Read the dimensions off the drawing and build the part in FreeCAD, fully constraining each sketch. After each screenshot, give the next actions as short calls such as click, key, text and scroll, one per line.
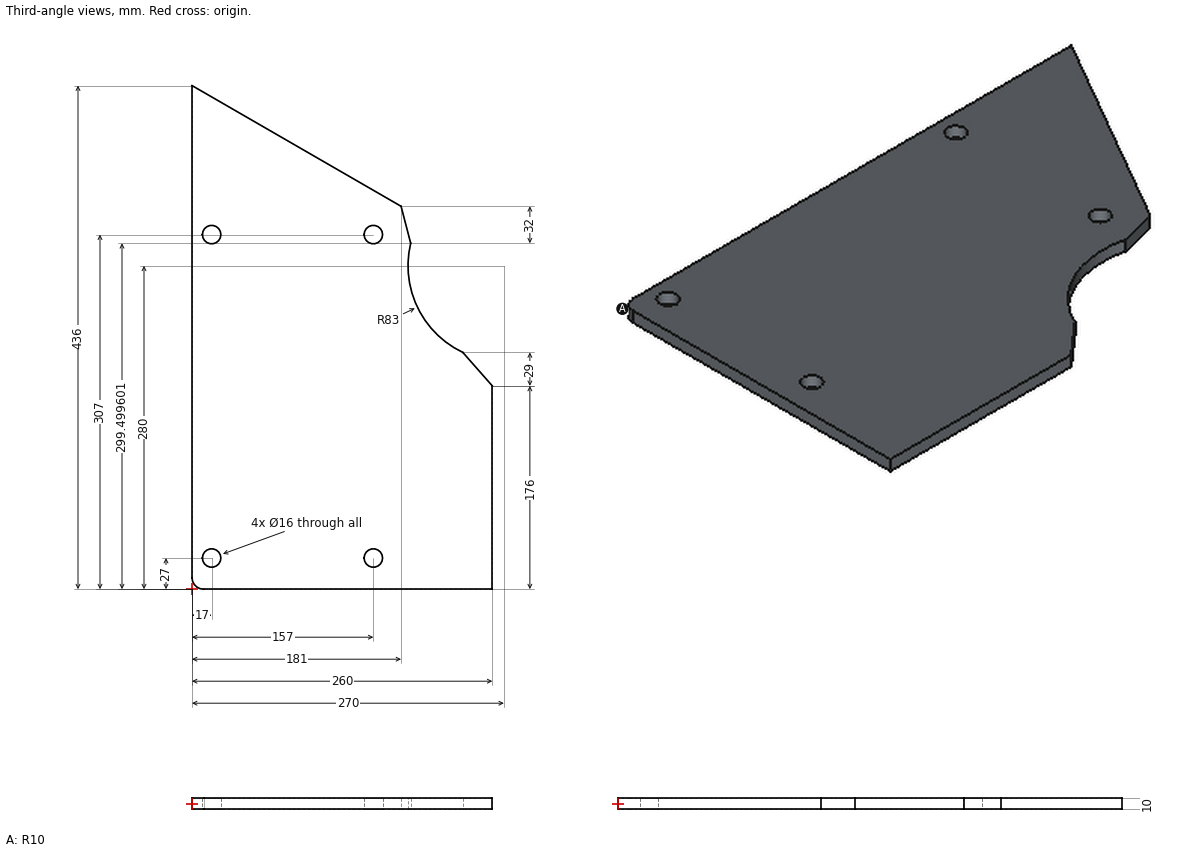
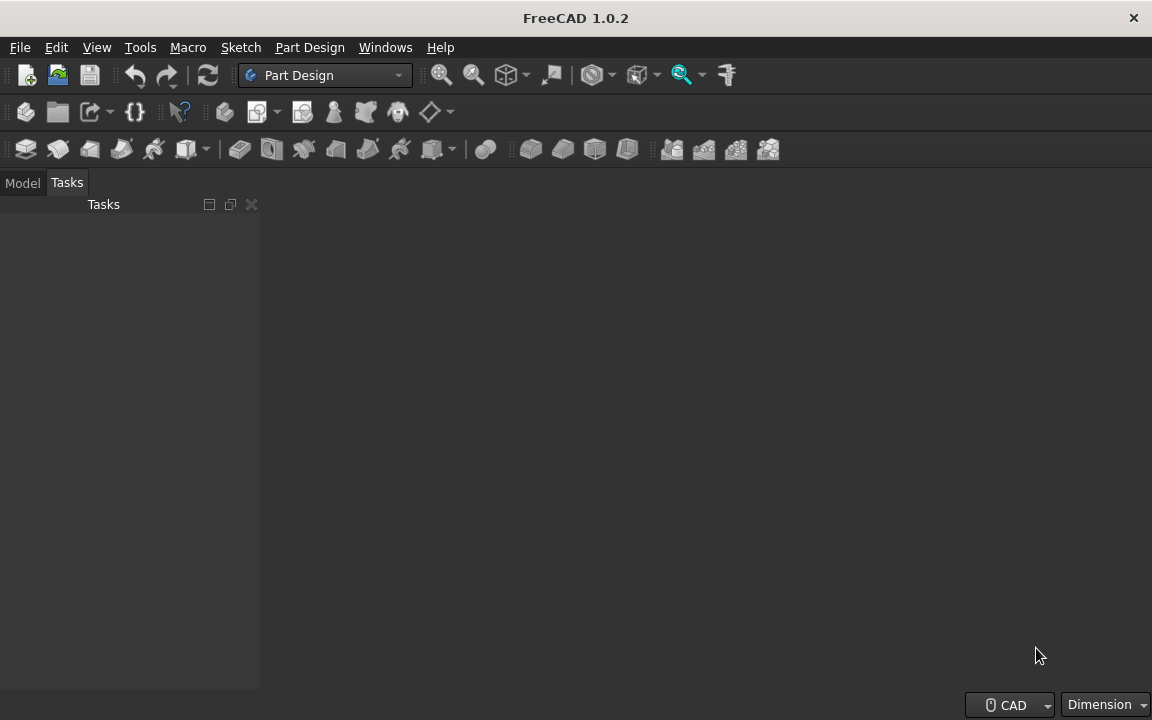
key(ctrl+n)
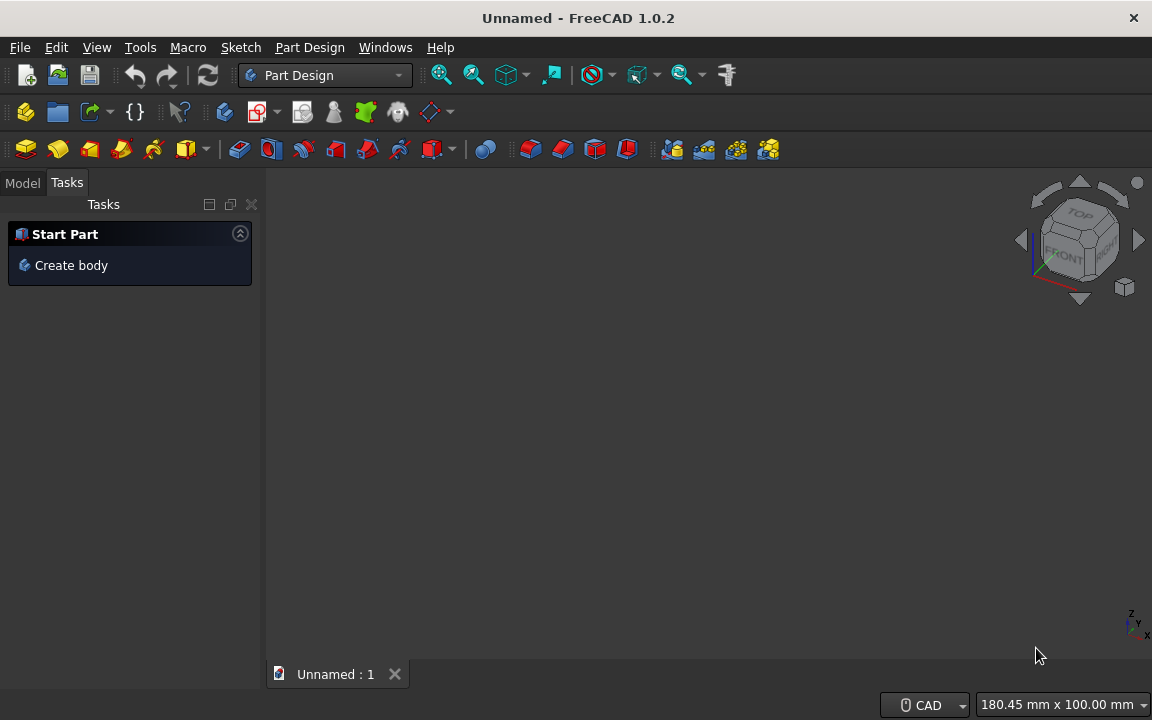
click(258, 112)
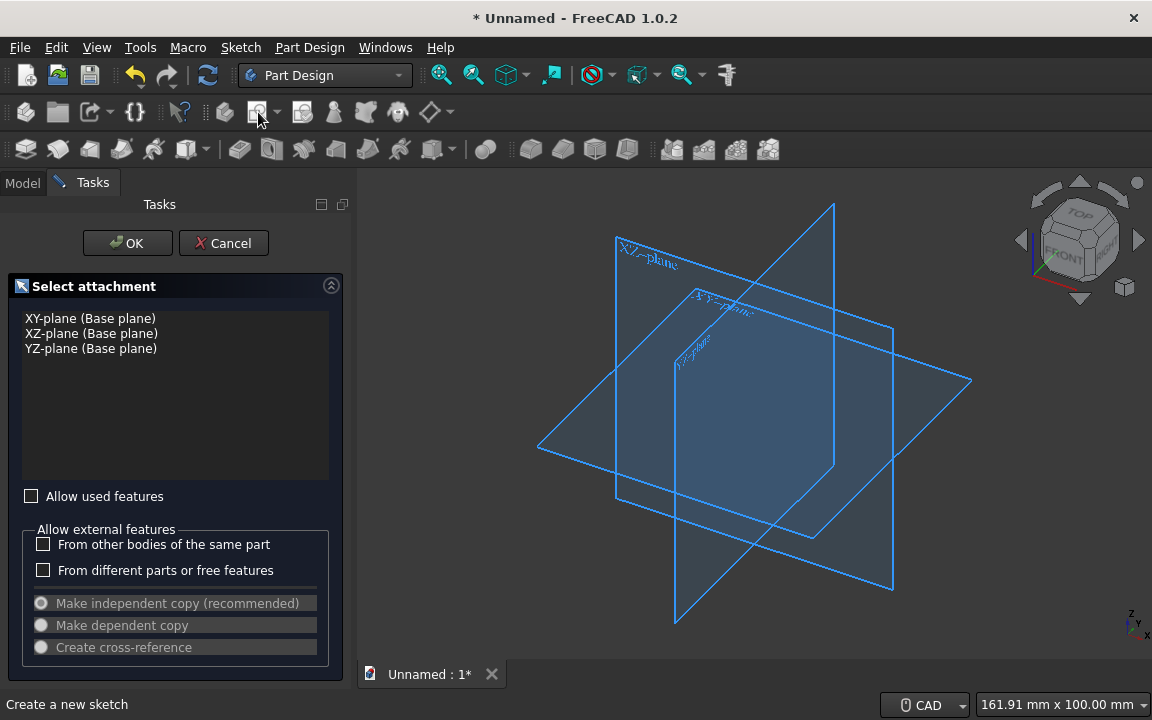
click(82, 318)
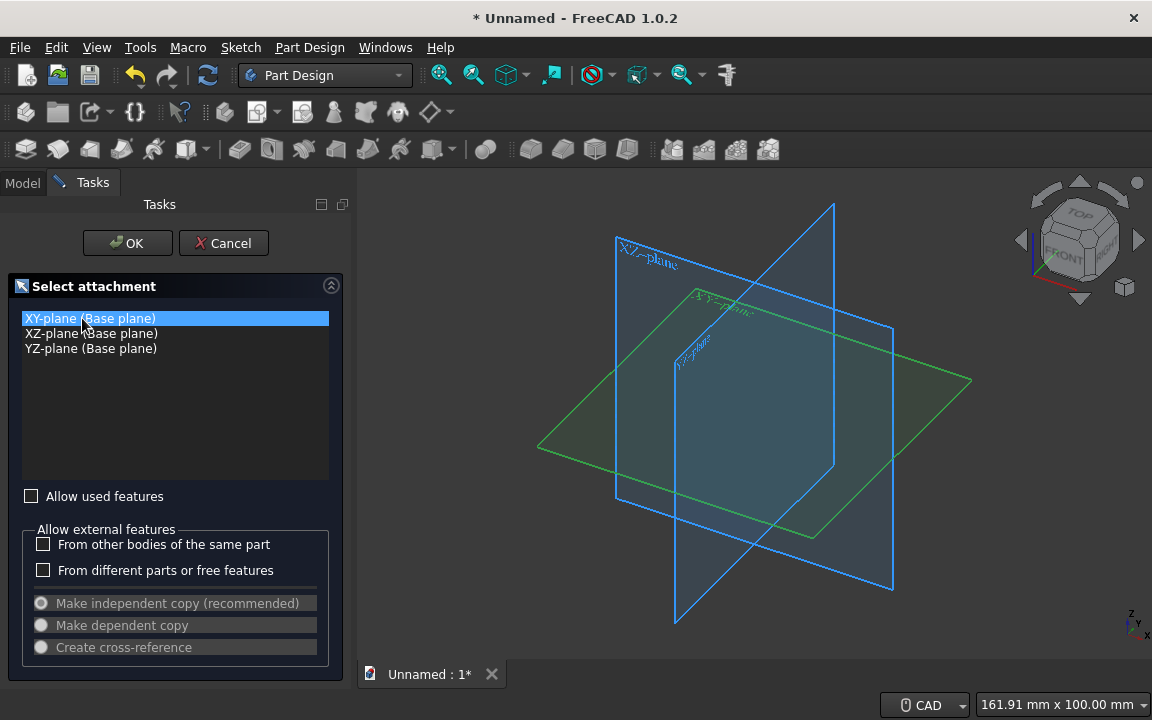
click(128, 243)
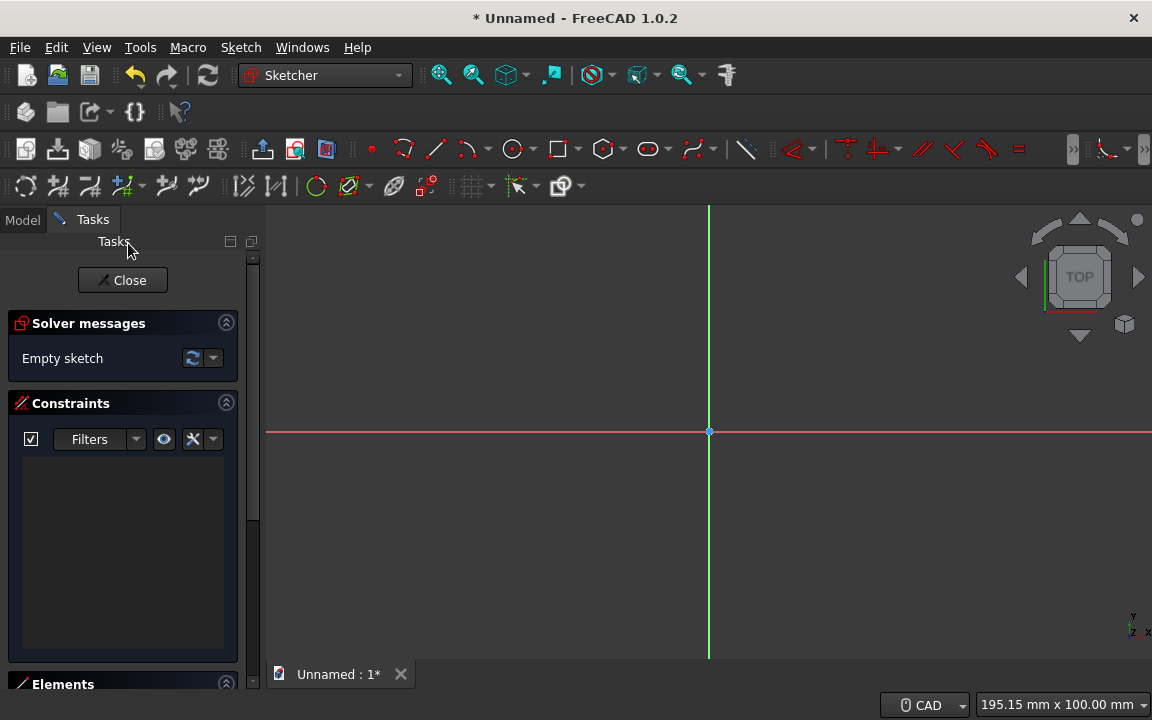
scroll(537, 587, down, 10)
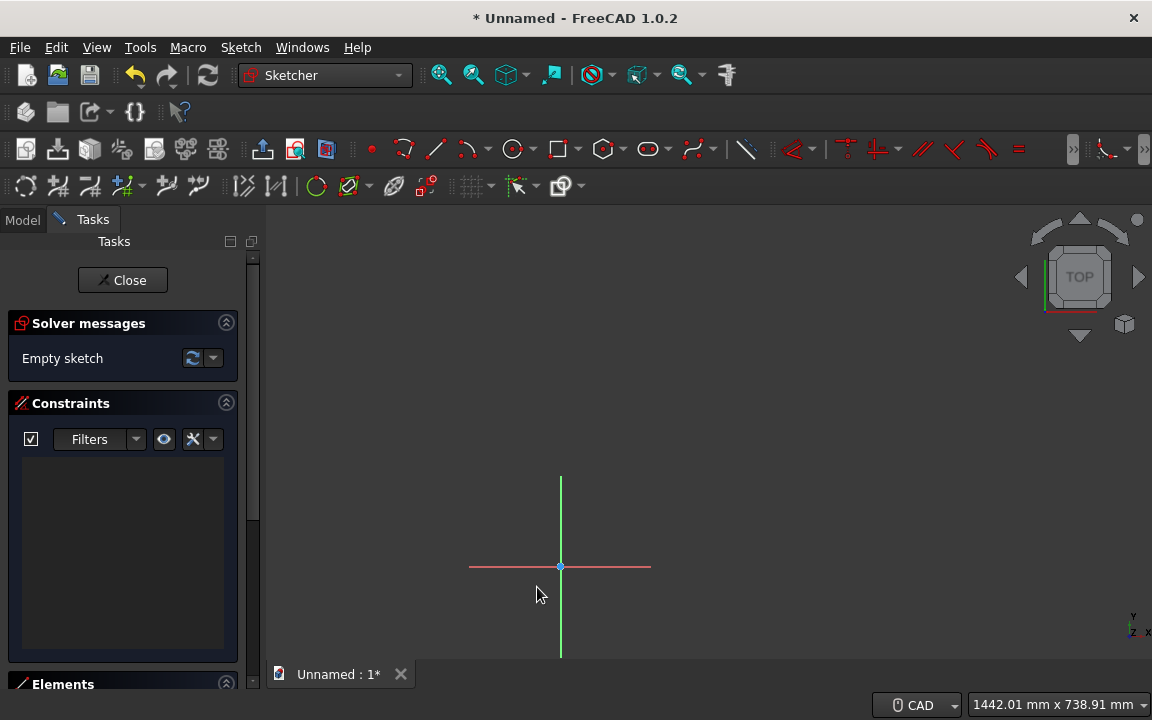
click(404, 150)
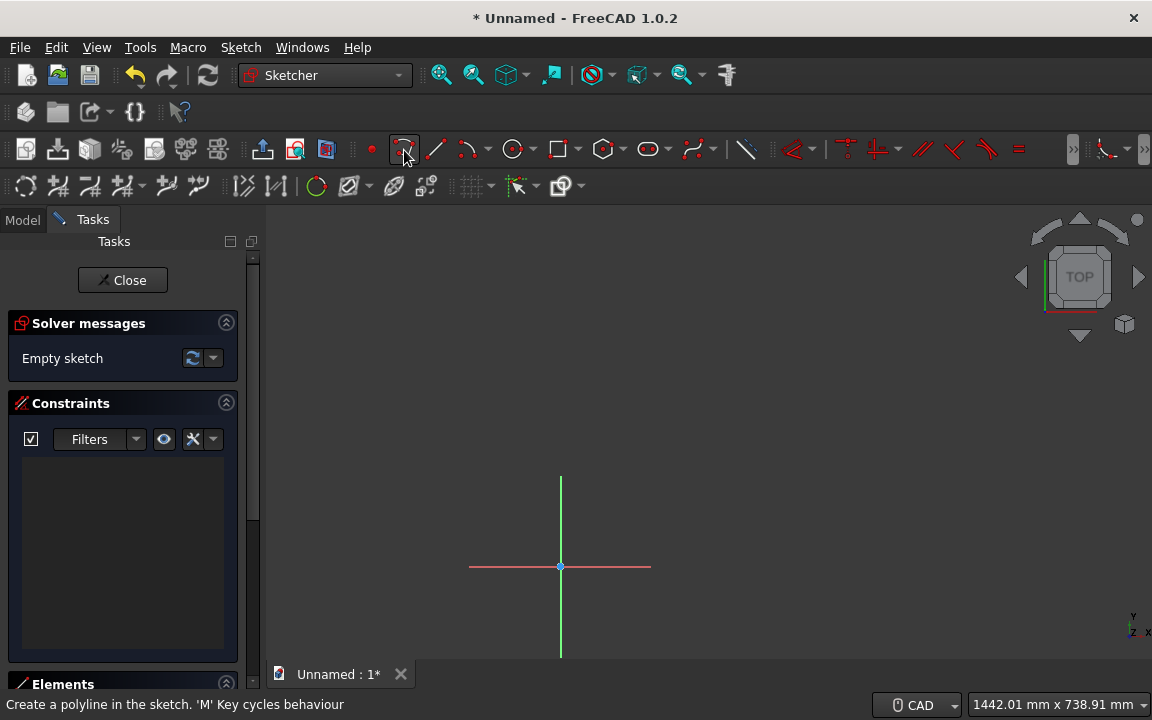
click(677, 383)
click(672, 363)
click(561, 299)
click(561, 567)
click(720, 558)
click(720, 459)
click(705, 441)
right_click(705, 441)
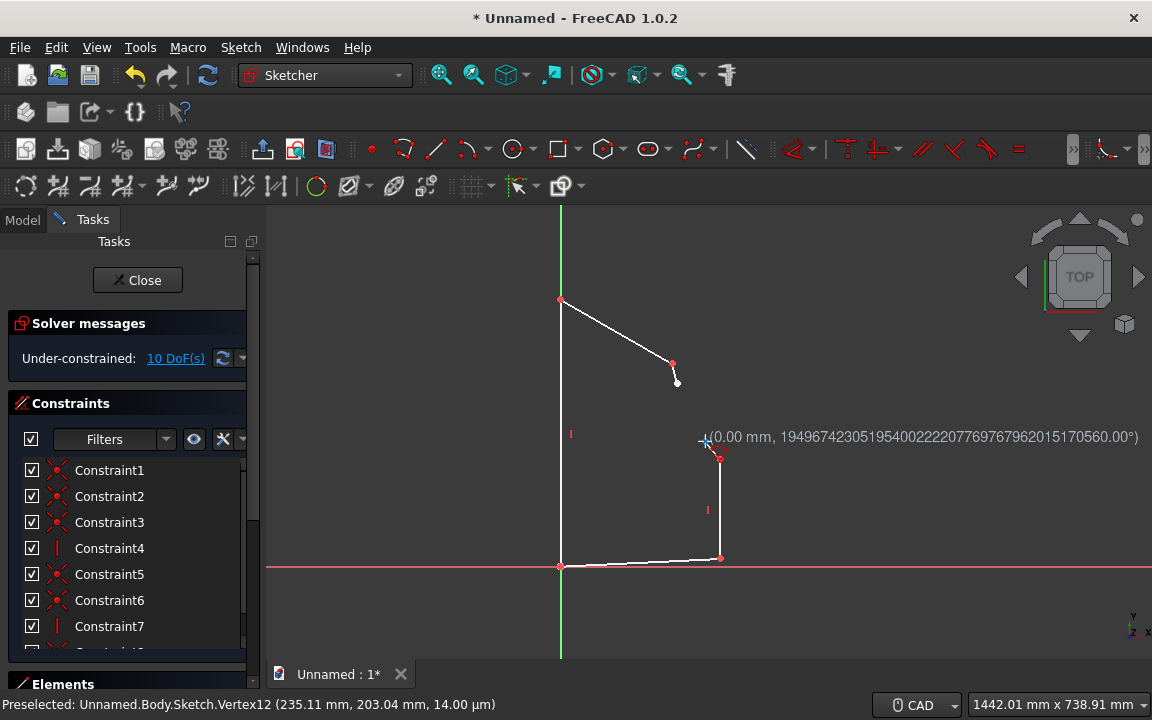
key(g)
key(3)
key(a)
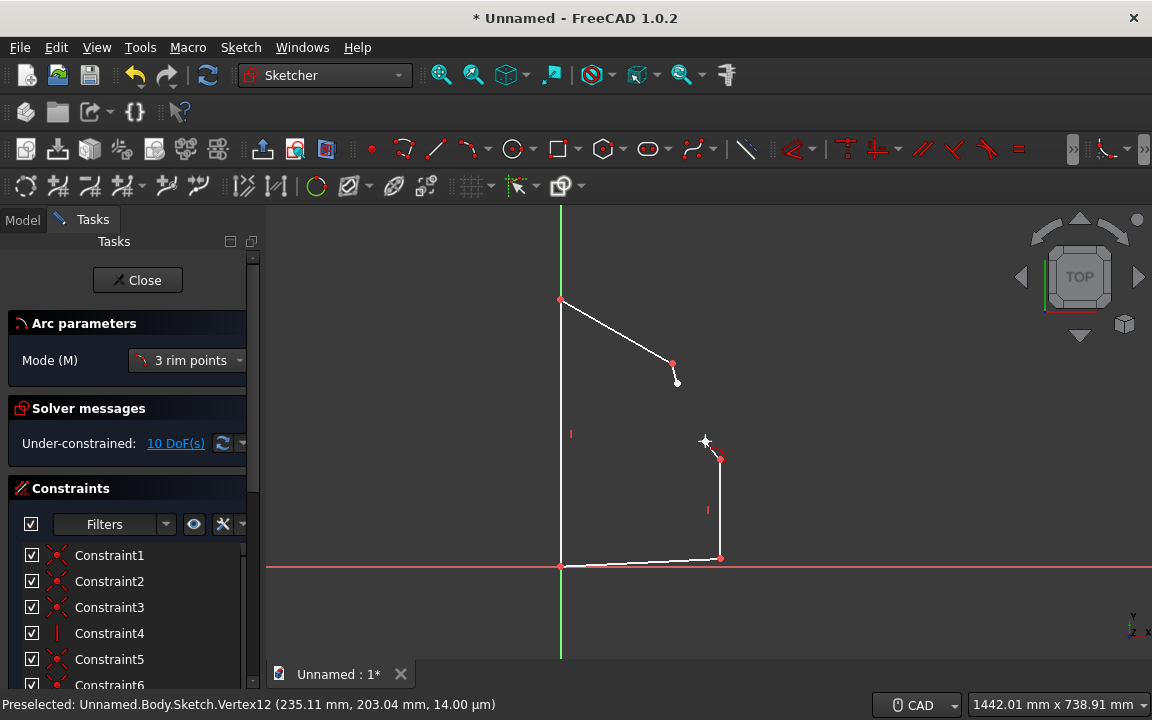
scroll(705, 441, up, 2)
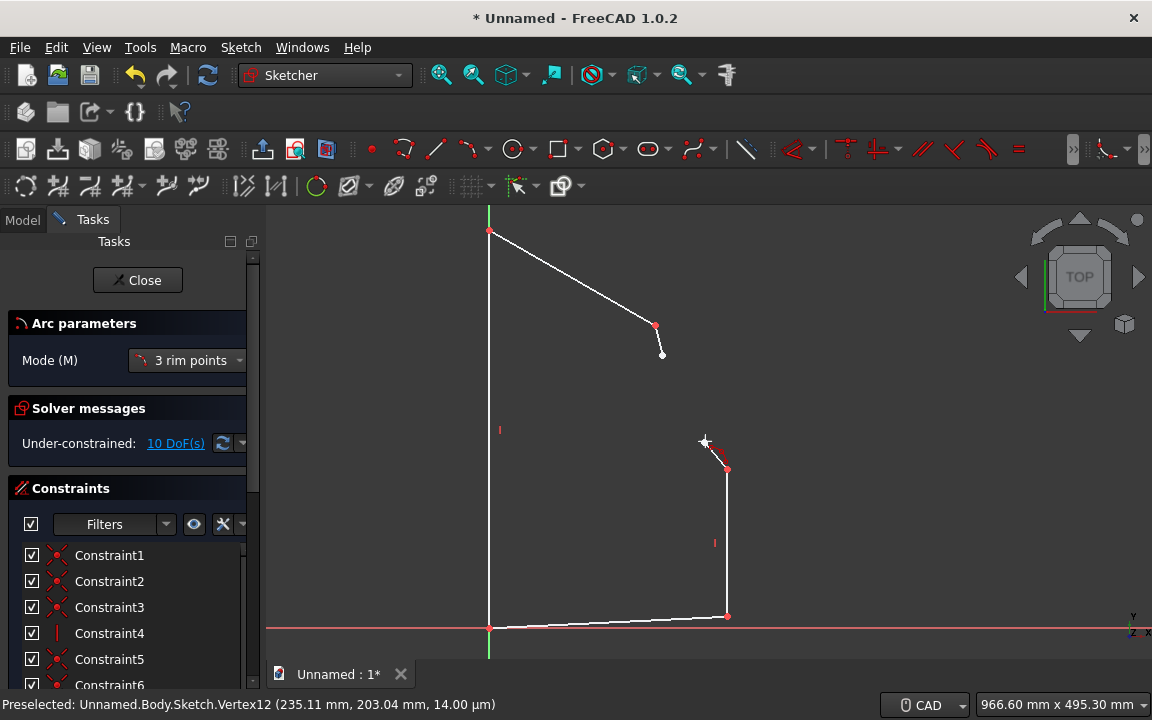
click(705, 442)
click(663, 356)
click(668, 404)
key(Escape)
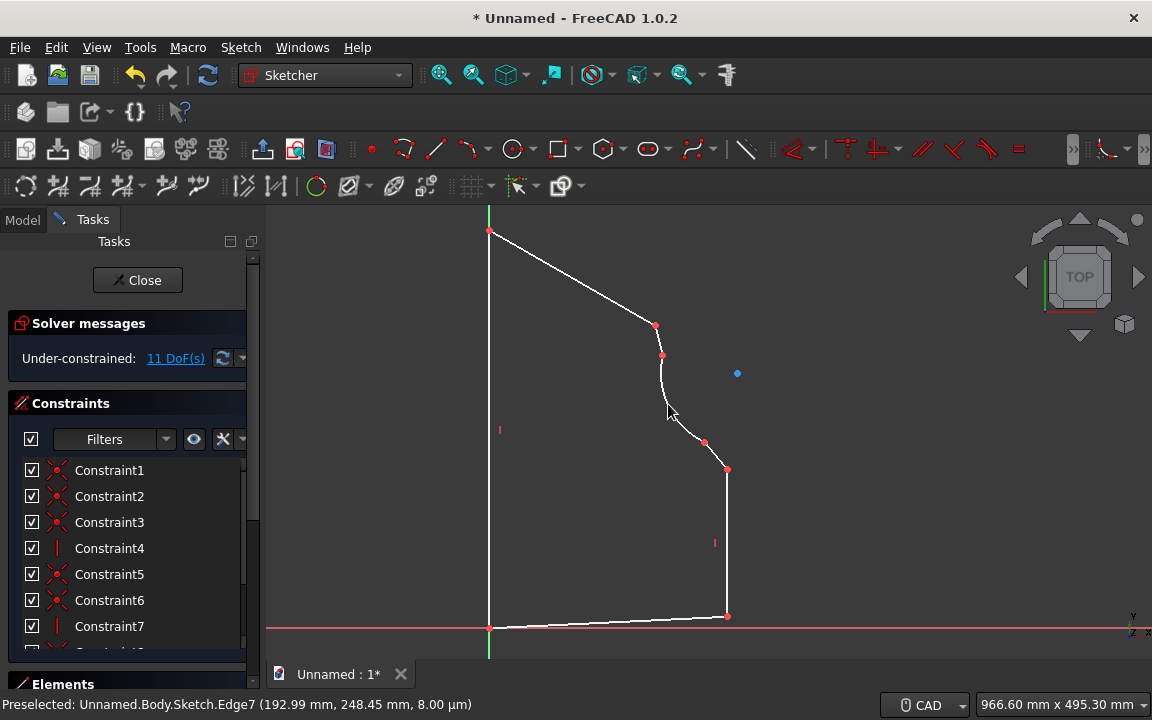
click(561, 625)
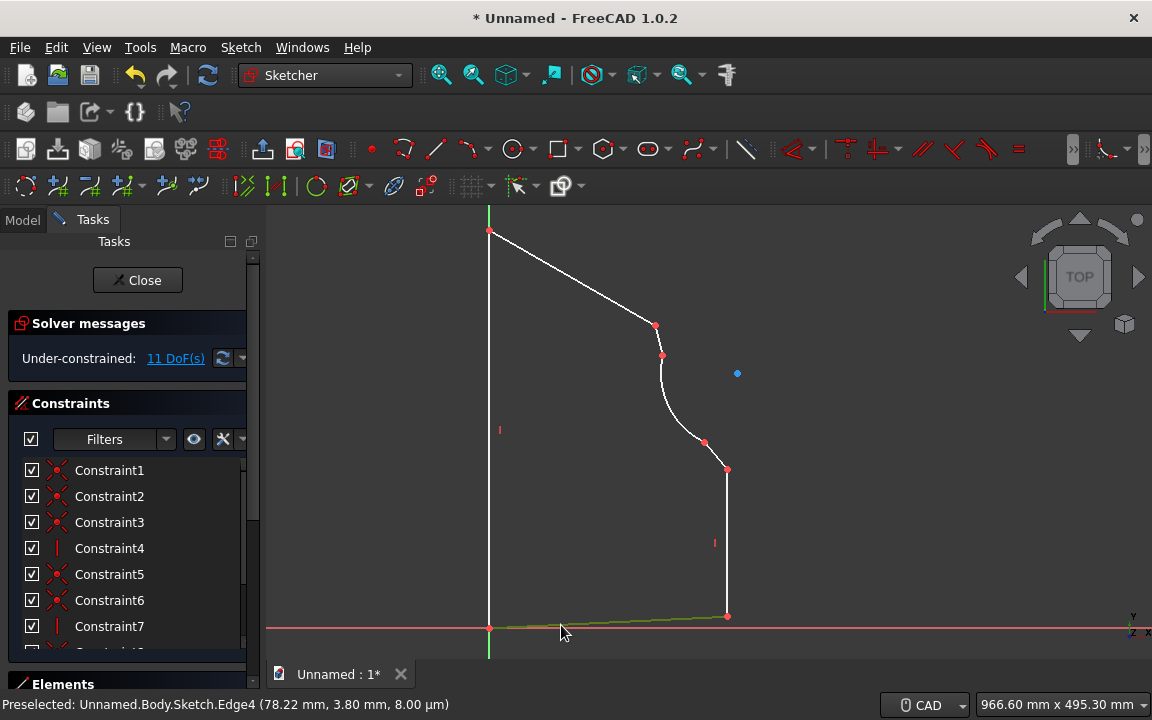
key(h)